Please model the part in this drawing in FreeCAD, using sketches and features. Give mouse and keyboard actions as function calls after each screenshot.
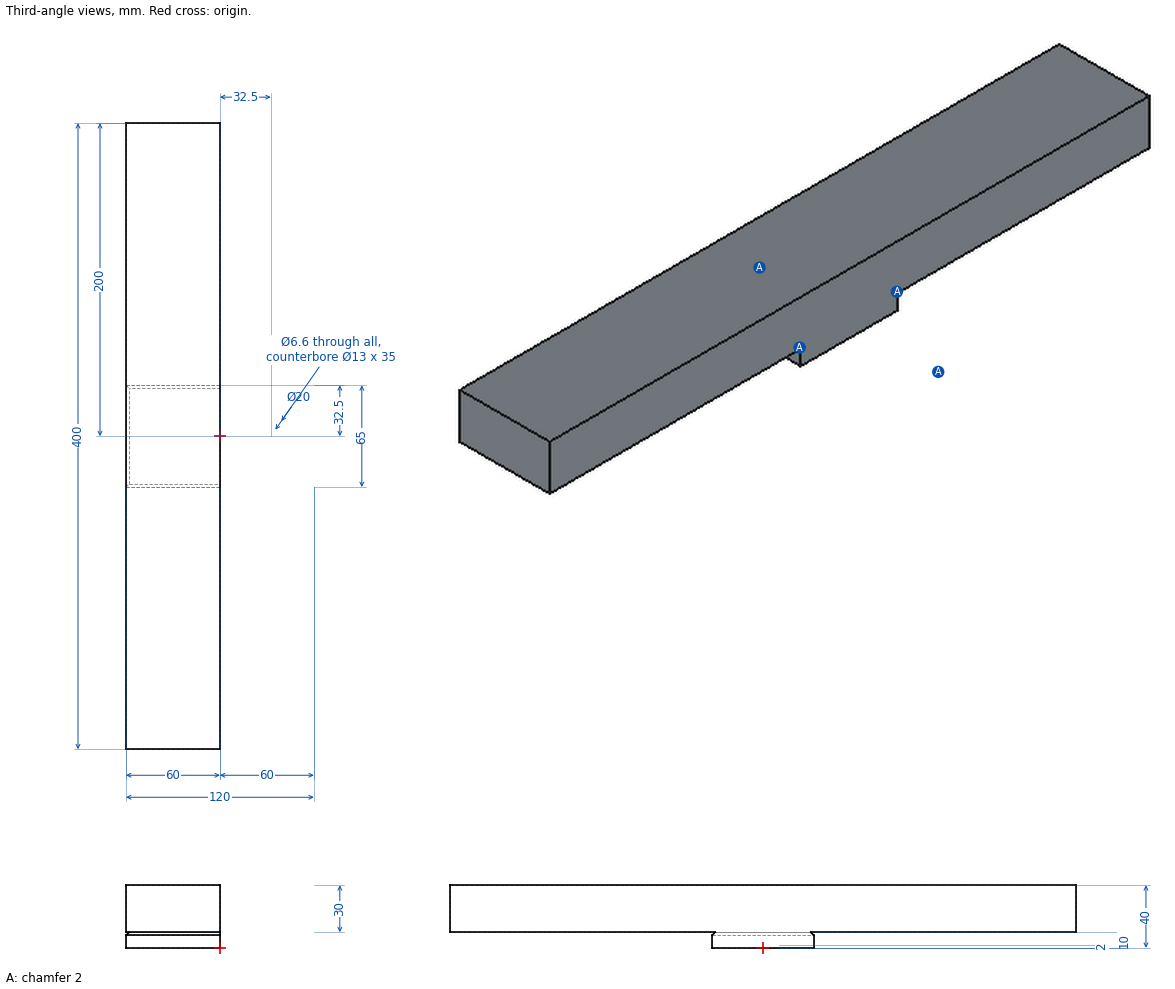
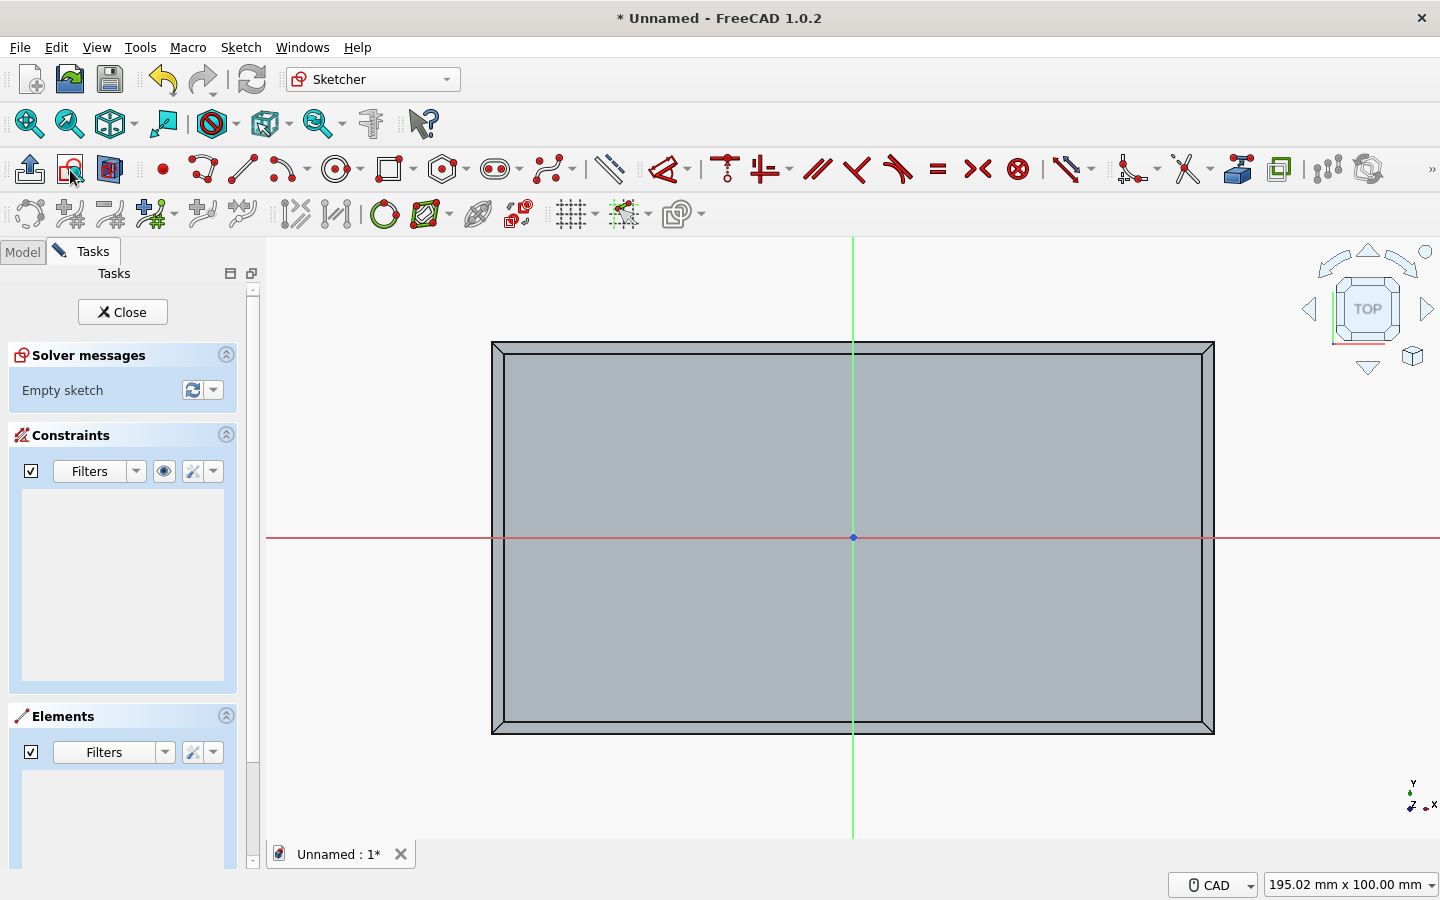
click(416, 170)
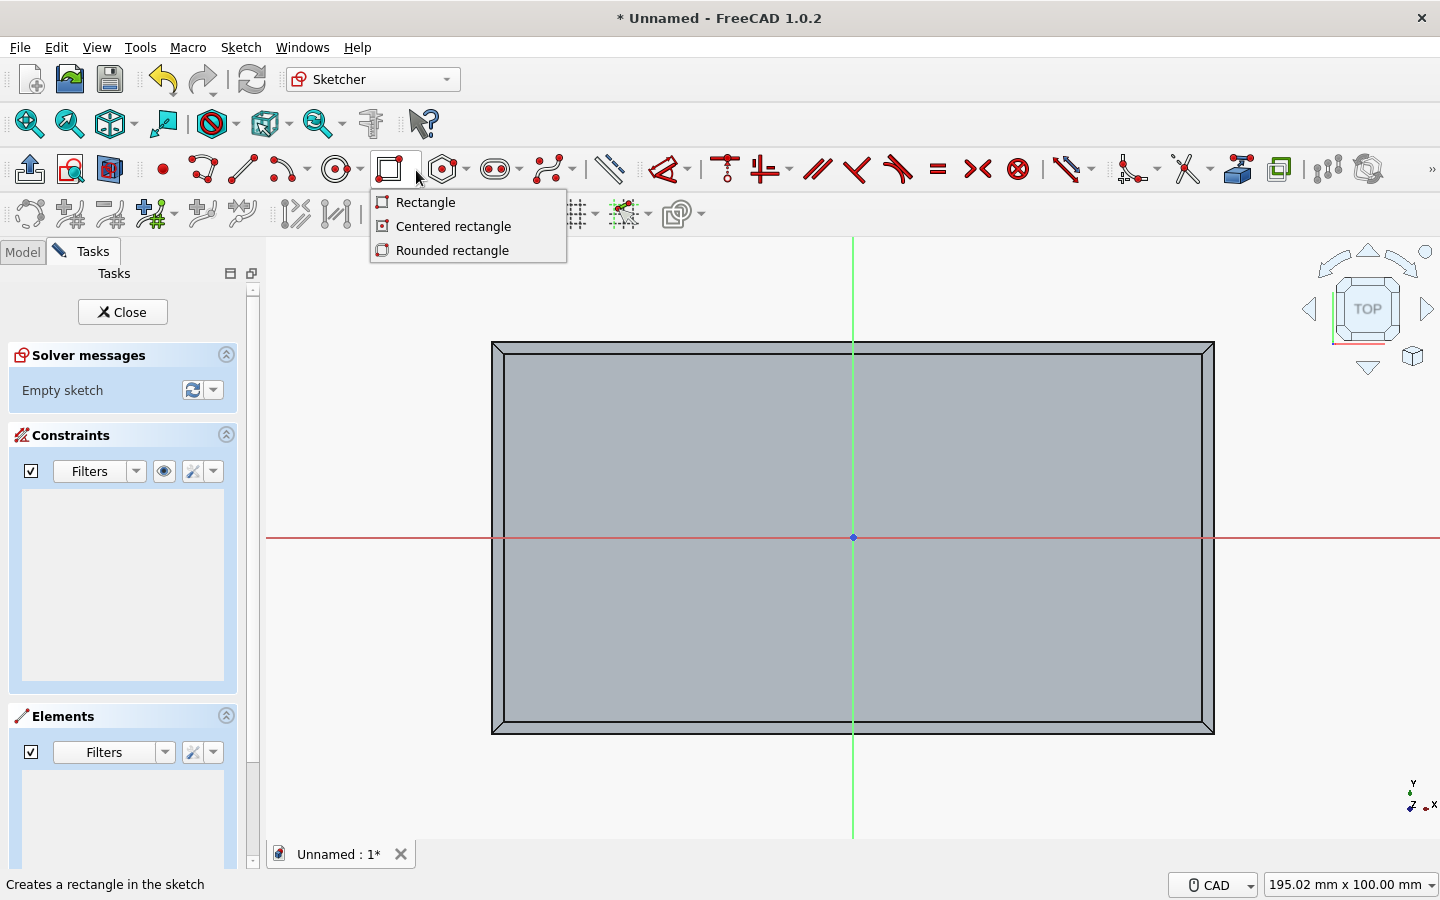
click(468, 226)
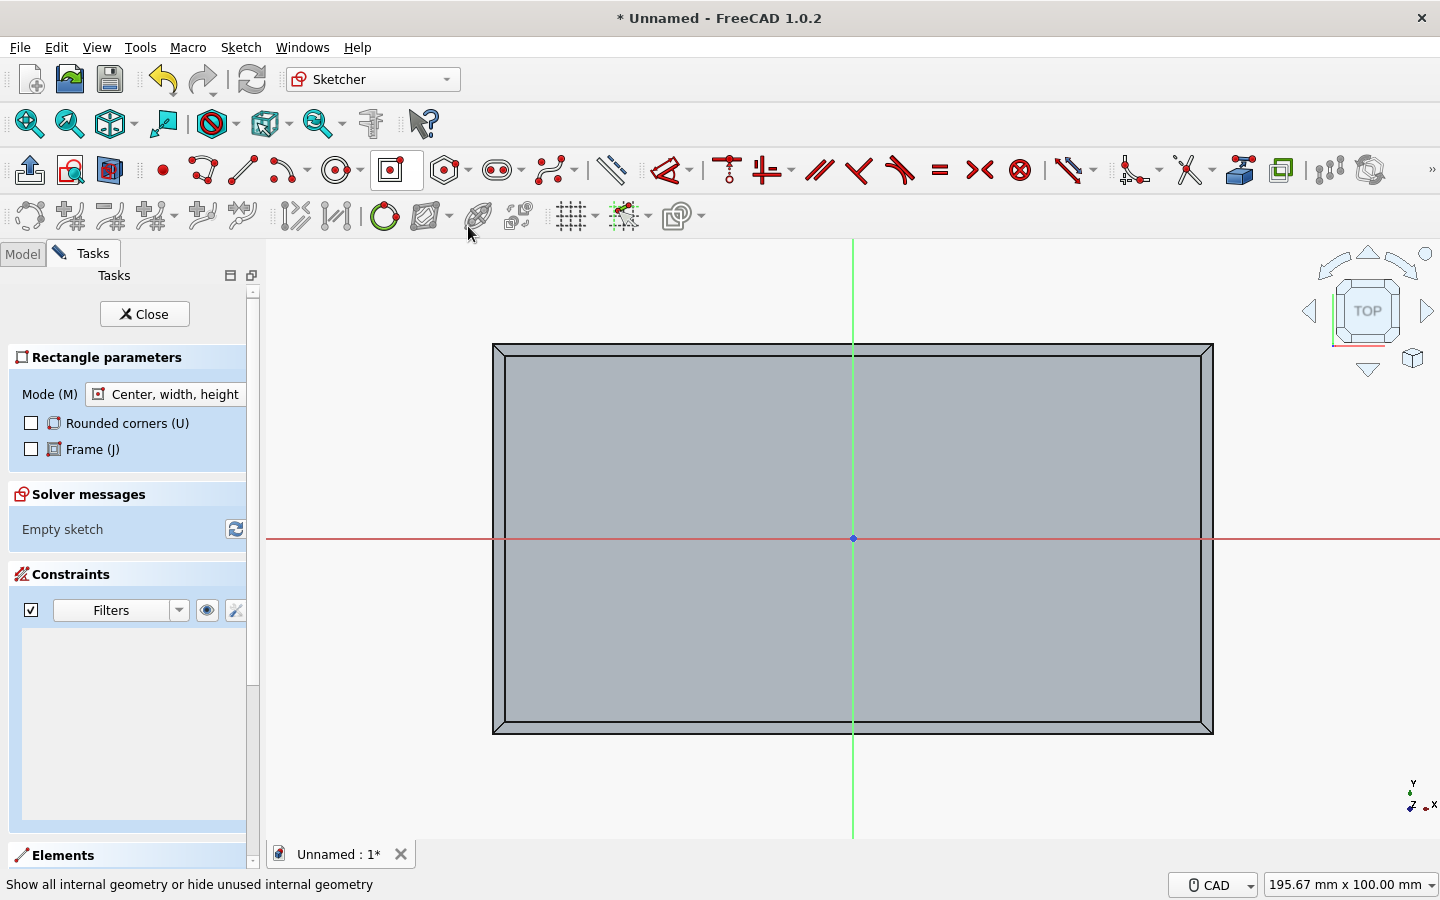
click(853, 539)
click(1213, 344)
key(Escape)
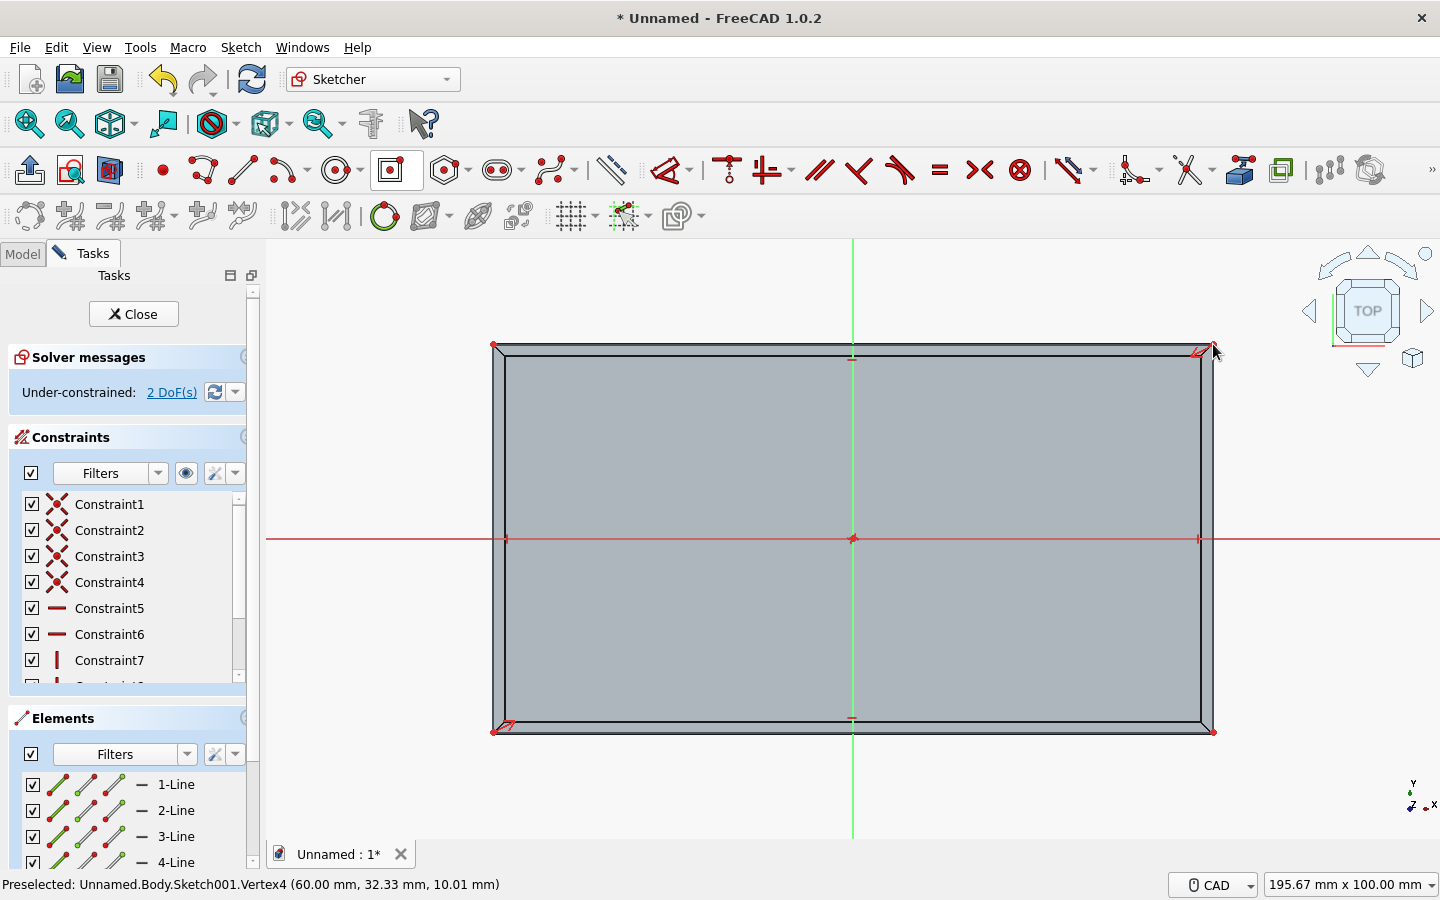
key(d)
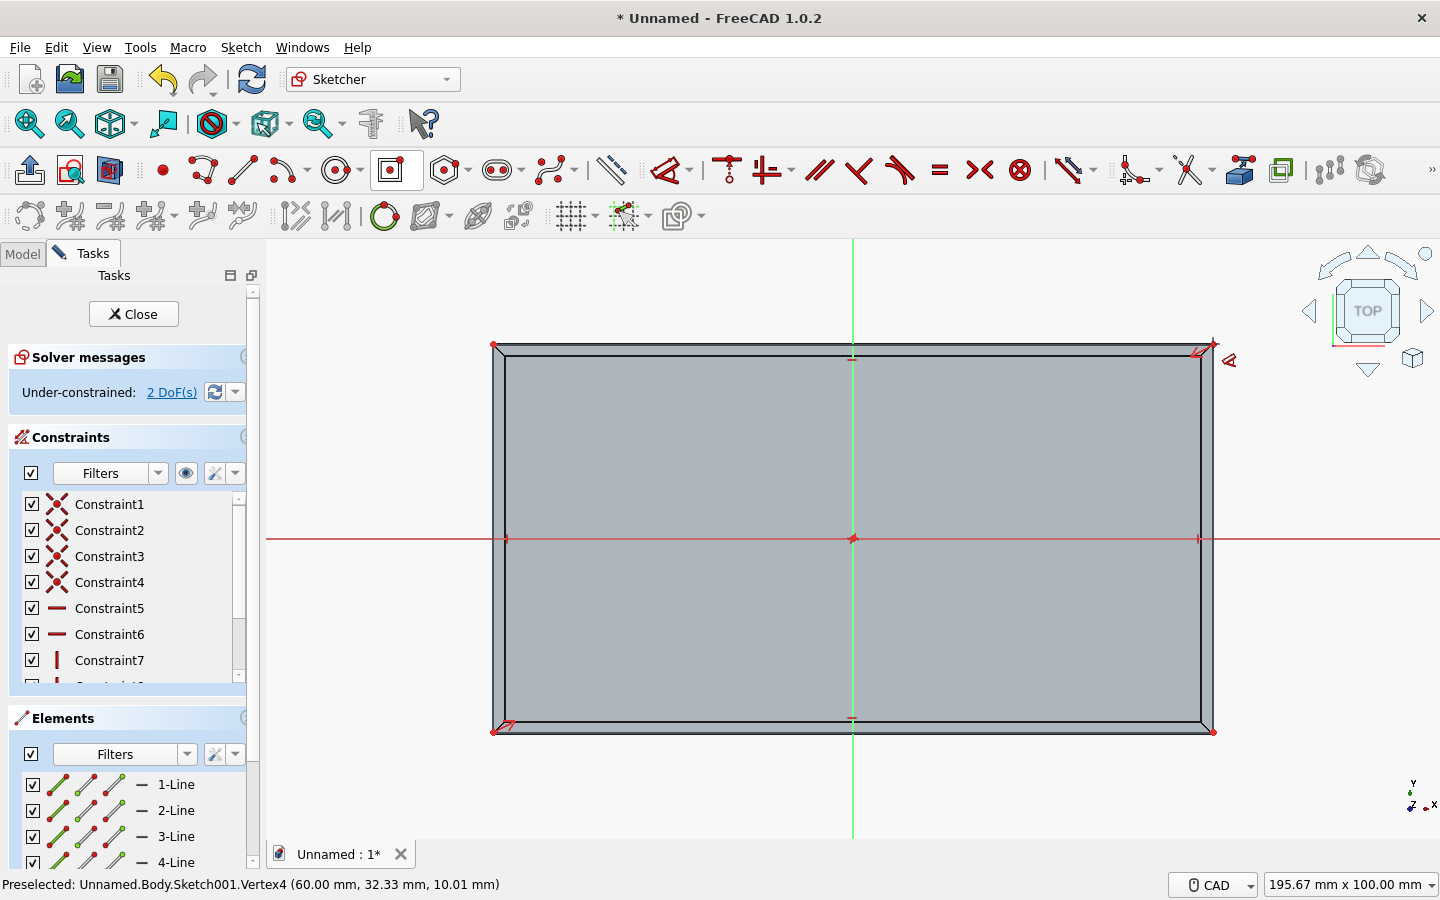
click(1213, 617)
click(1247, 450)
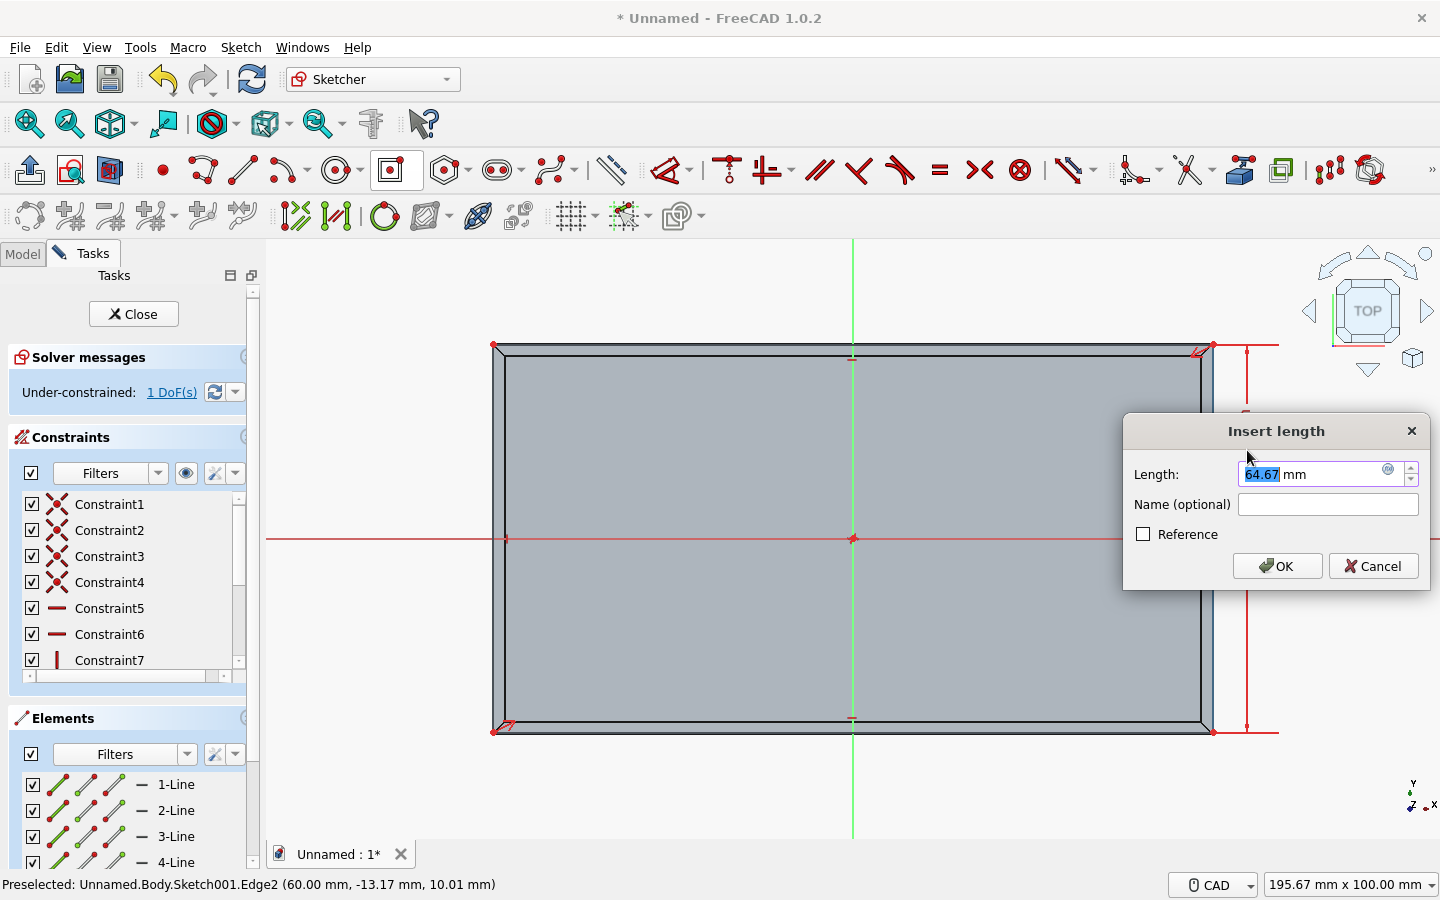
text(65)
key(Return)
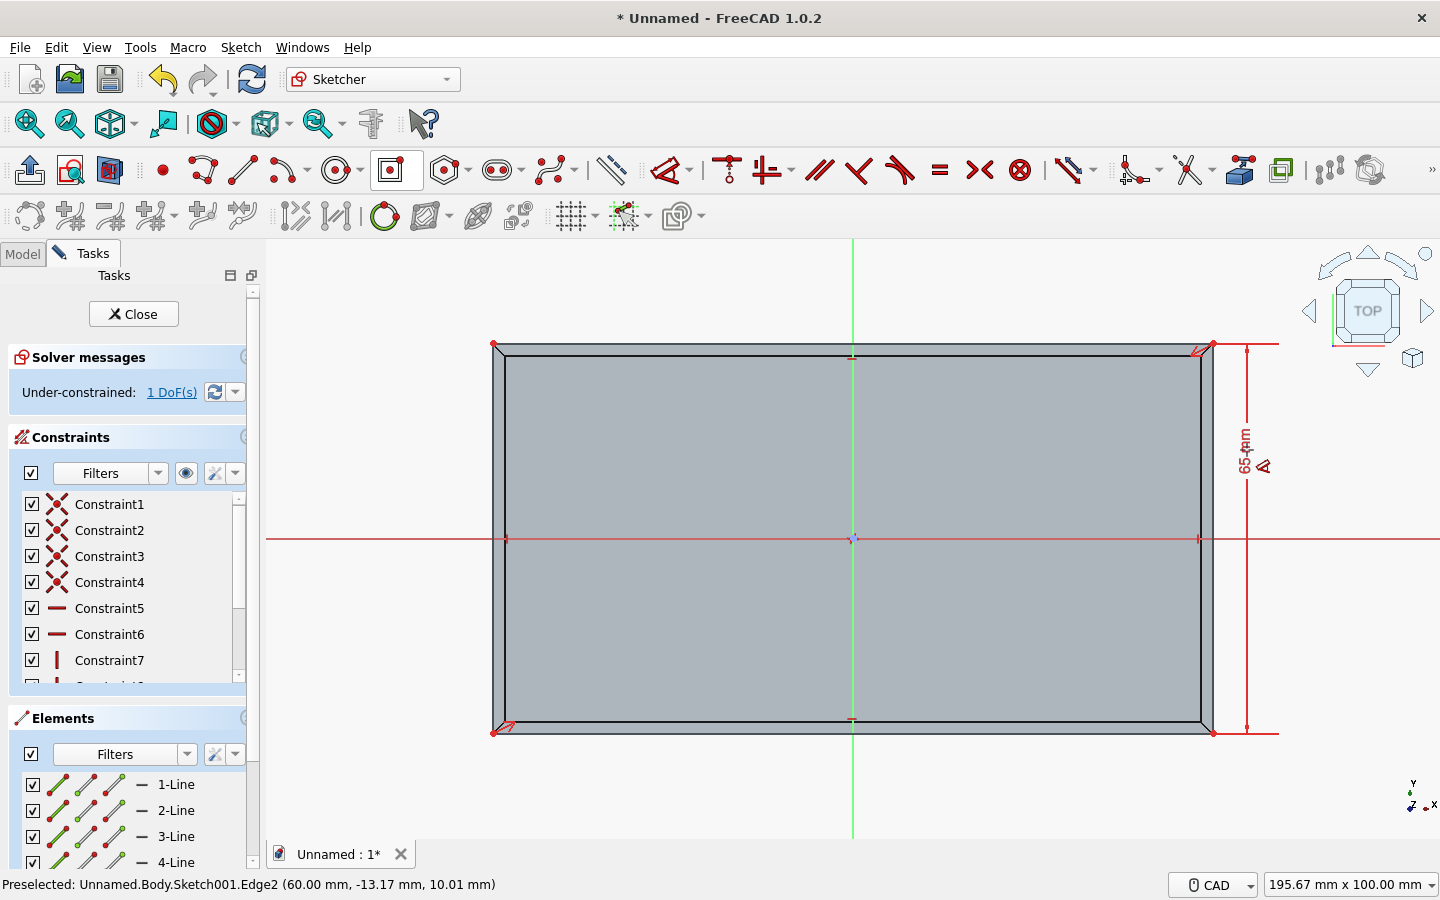
click(709, 734)
click(687, 768)